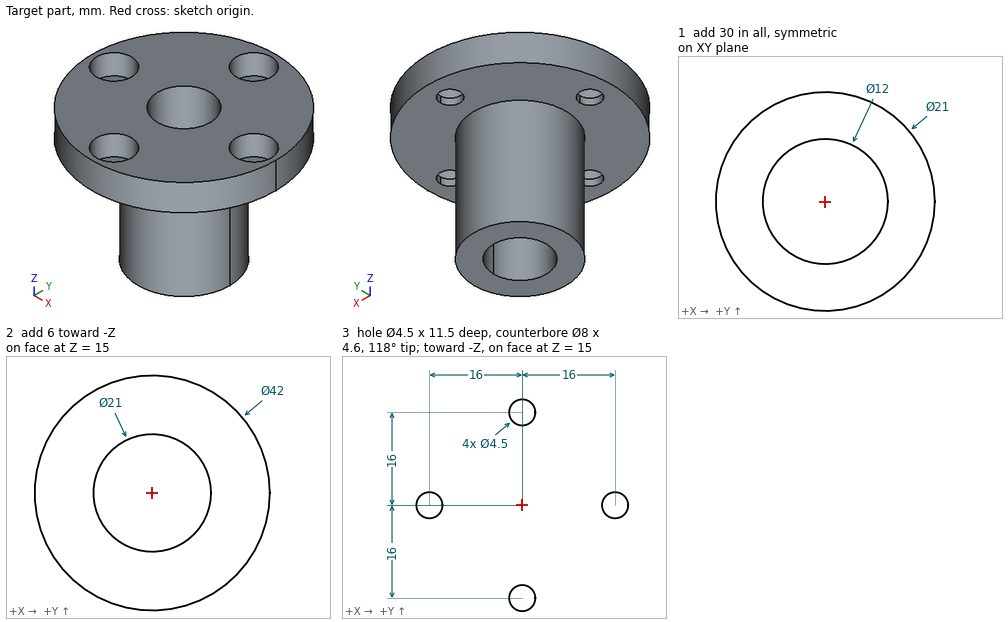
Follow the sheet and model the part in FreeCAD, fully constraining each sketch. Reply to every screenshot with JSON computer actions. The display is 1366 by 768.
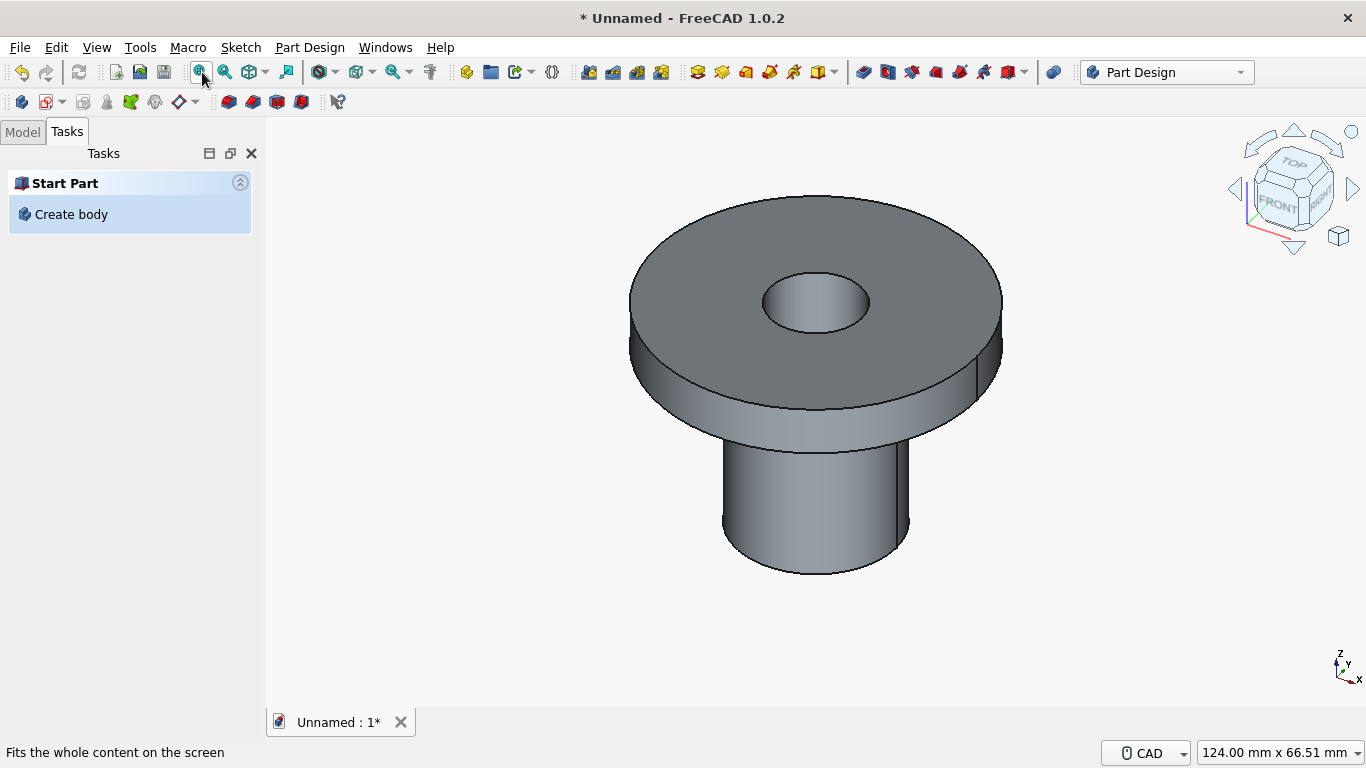
{"action": "left_click", "coordinate": [750, 245]}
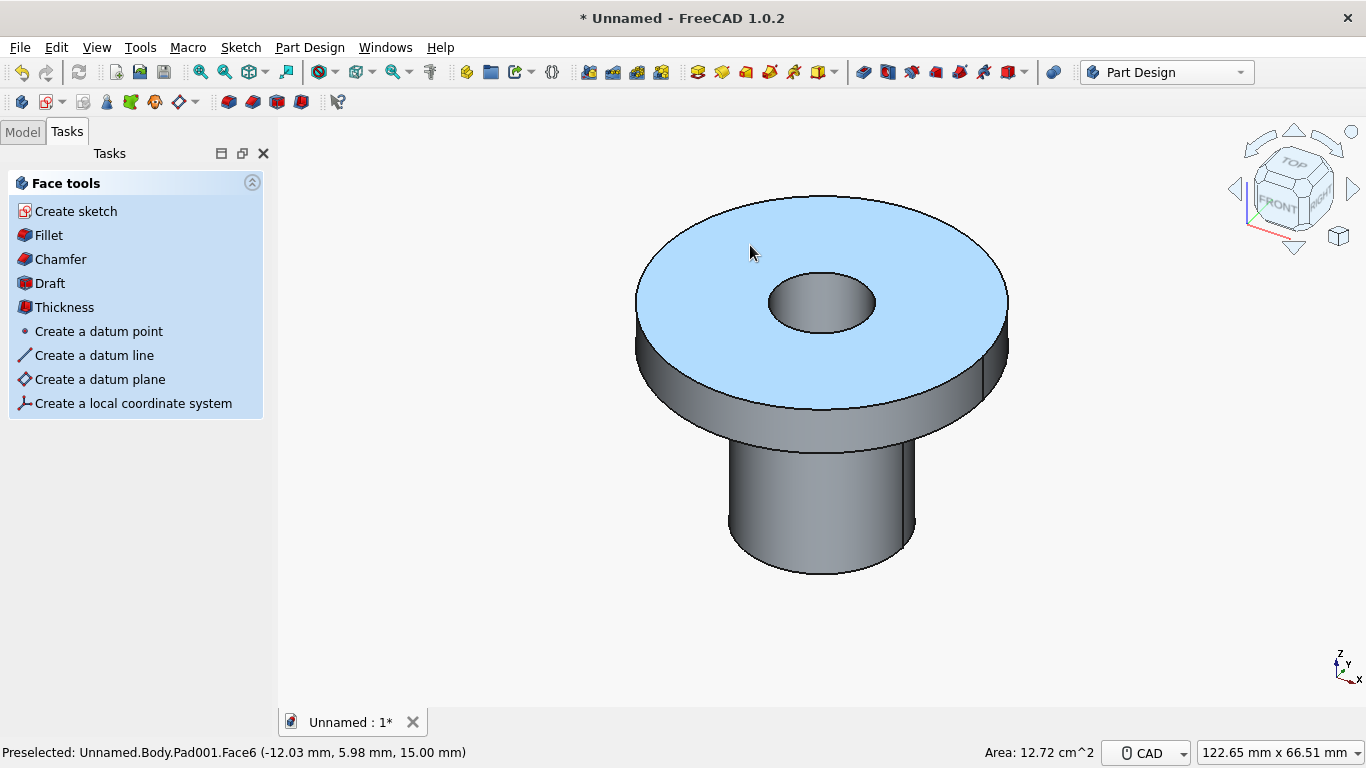
{"action": "left_click", "coordinate": [46, 102]}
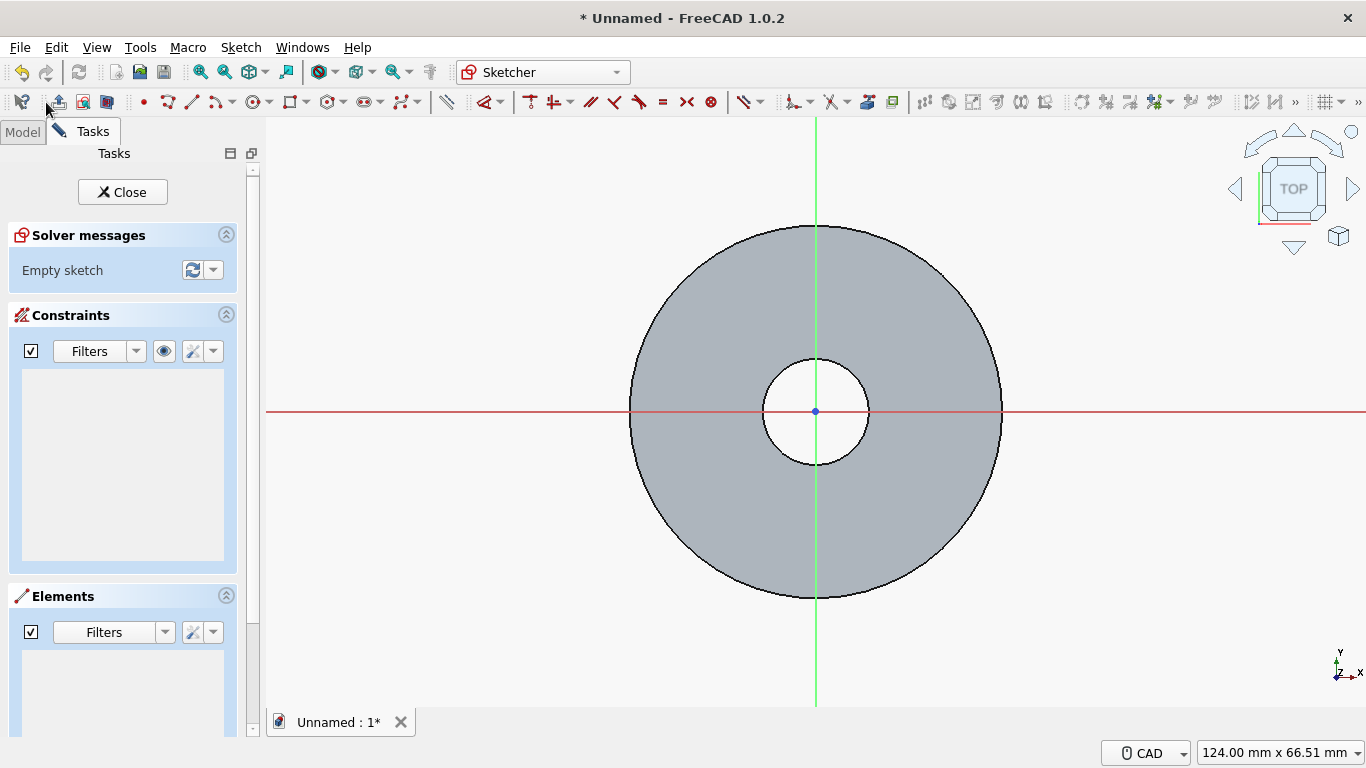
{"action": "left_click", "coordinate": [254, 102]}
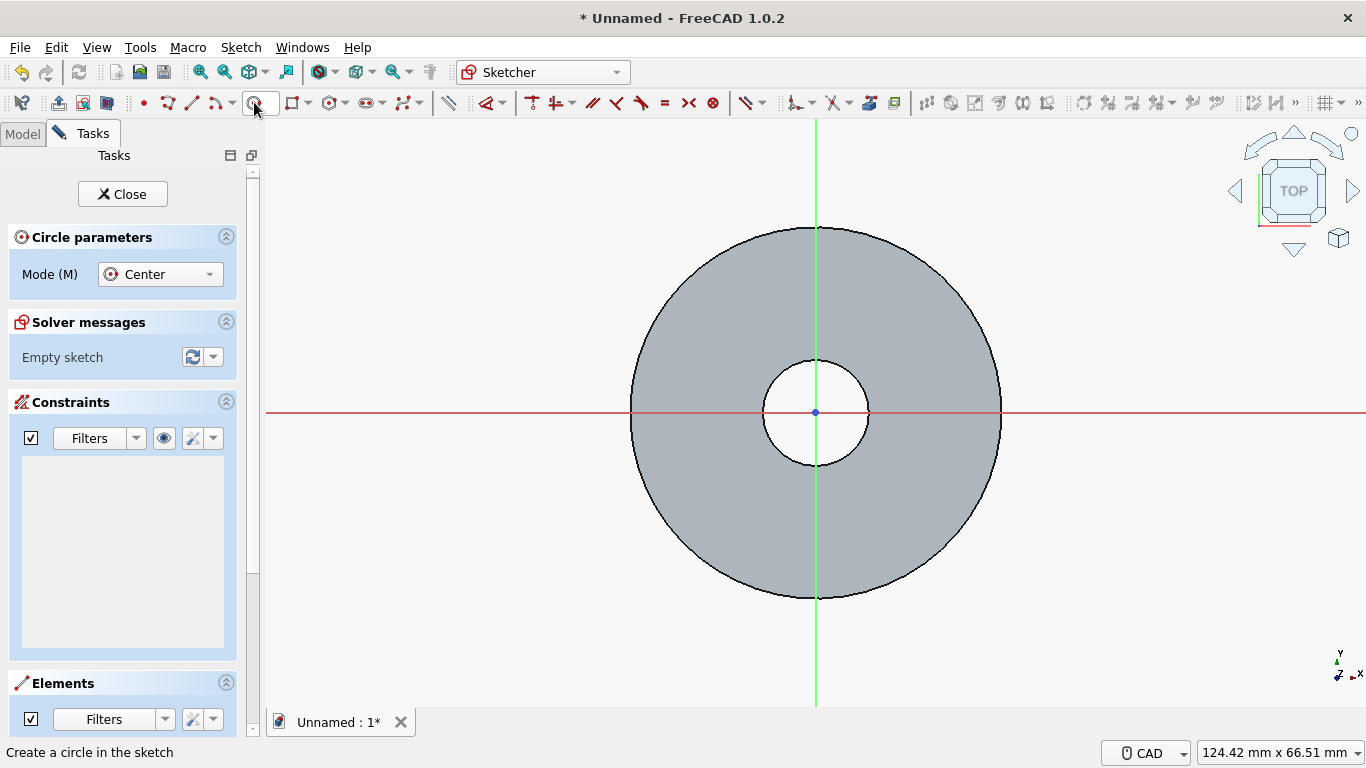
{"action": "left_click", "coordinate": [816, 272]}
{"action": "mouse_move", "coordinate": [830, 257]}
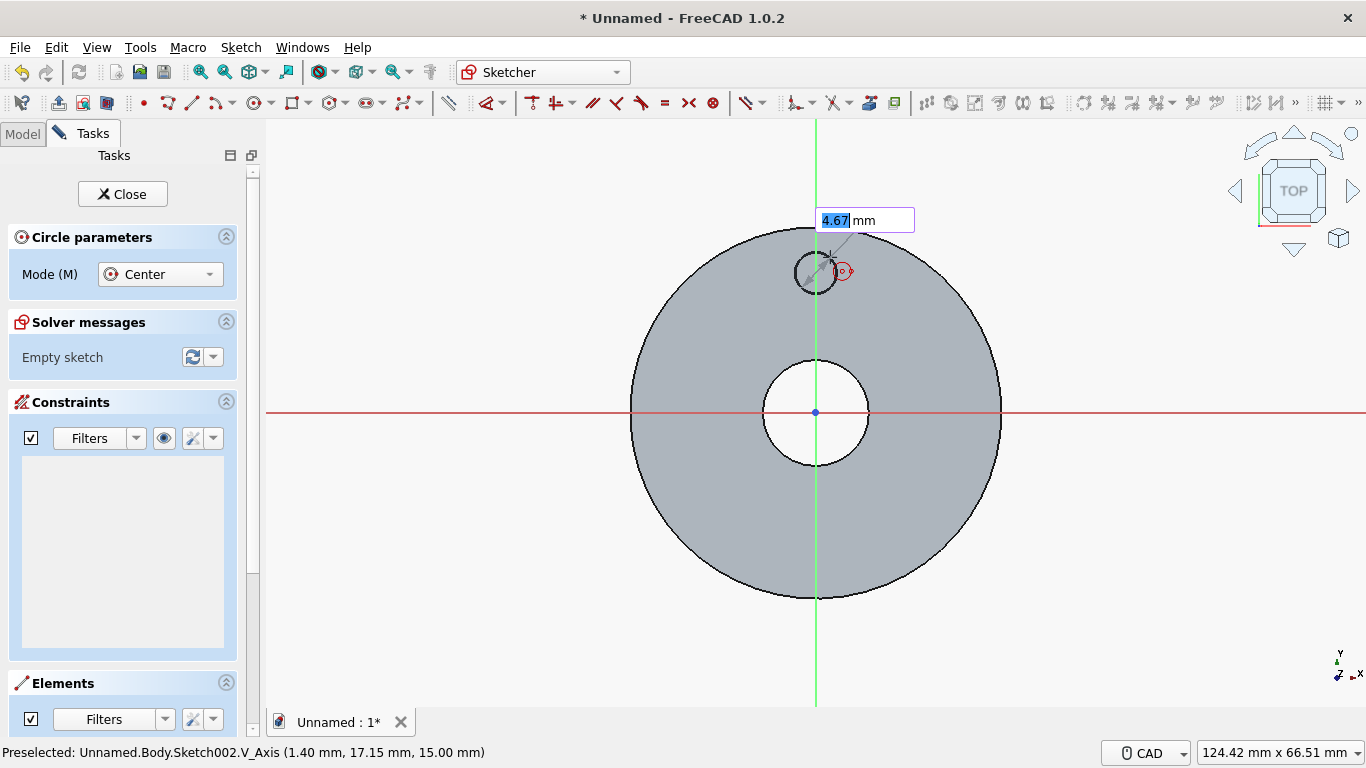
{"action": "type", "text": "4.5"}
{"action": "key", "text": "Return"}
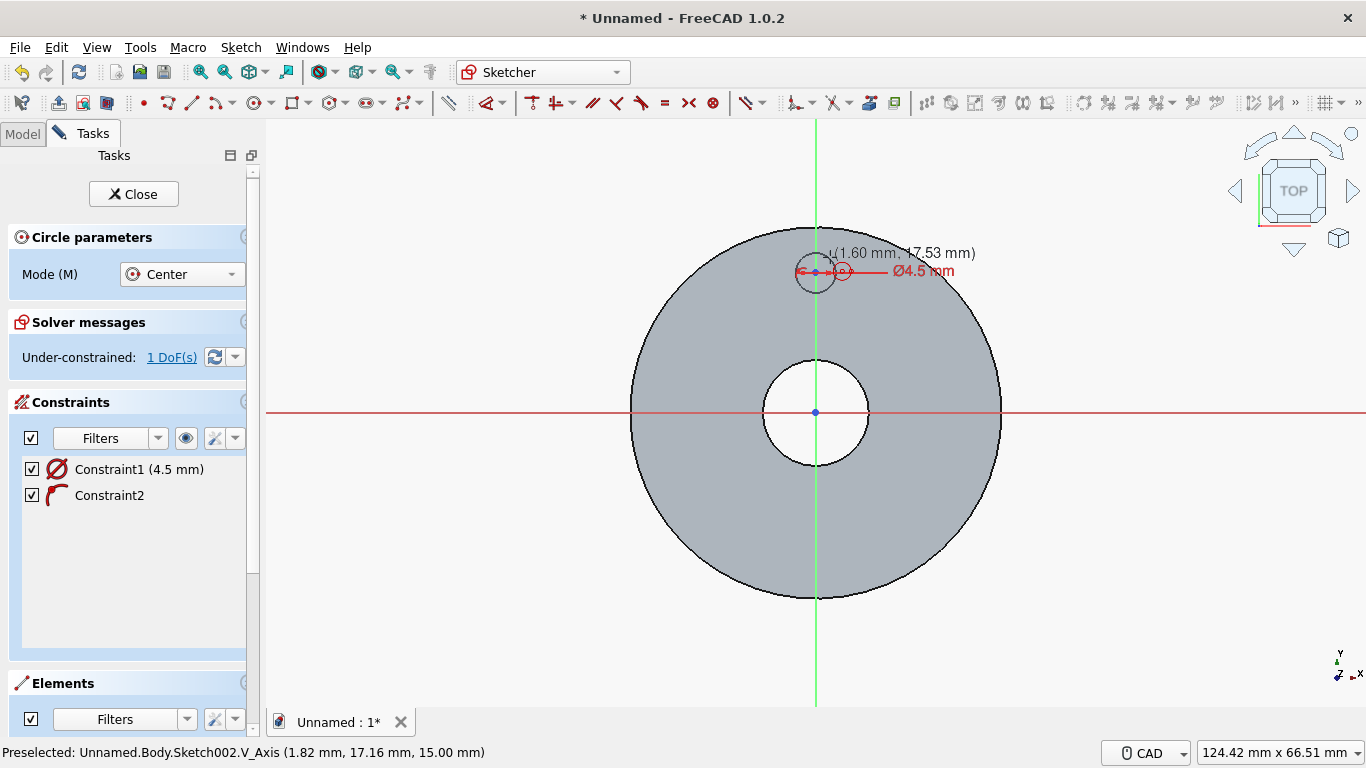
{"action": "left_click", "coordinate": [957, 413]}
{"action": "mouse_move", "coordinate": [971, 399]}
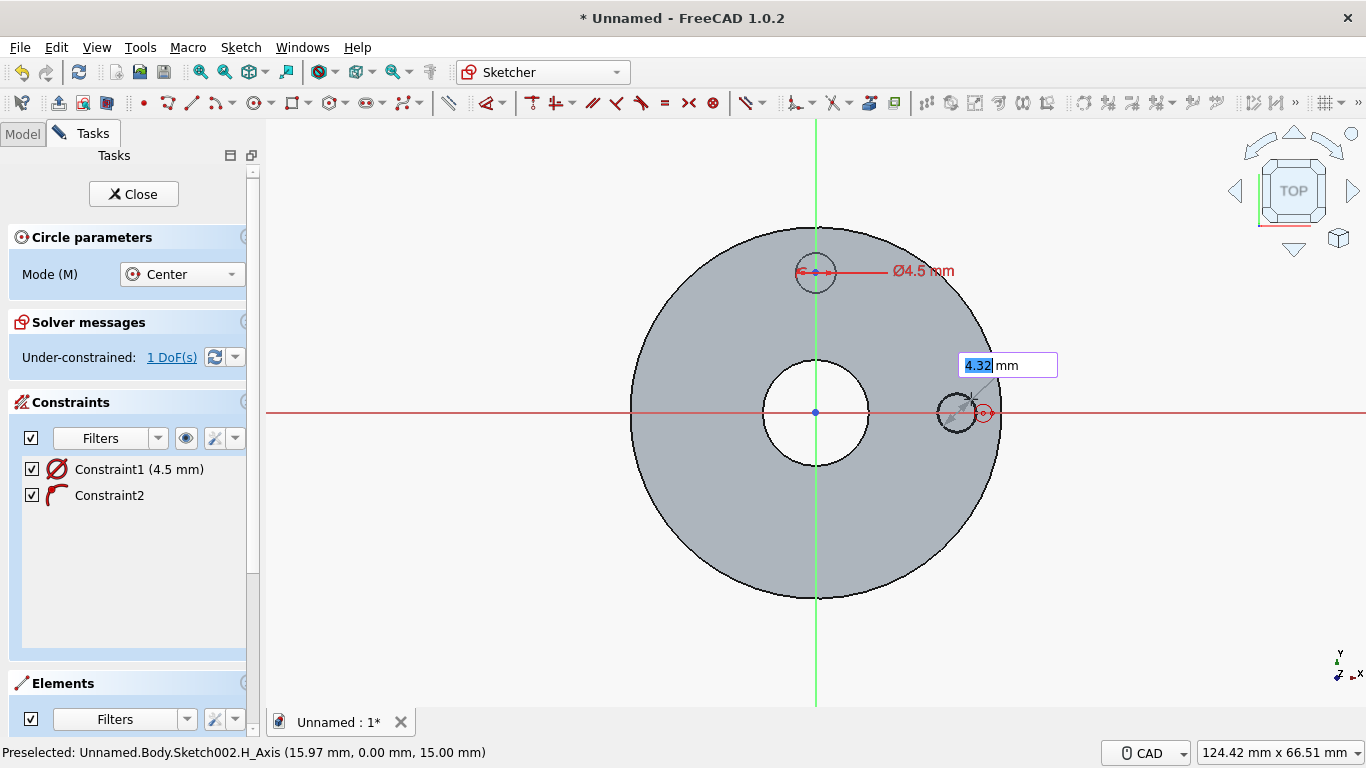
{"action": "type", "text": "4.5"}
{"action": "key", "text": "Return"}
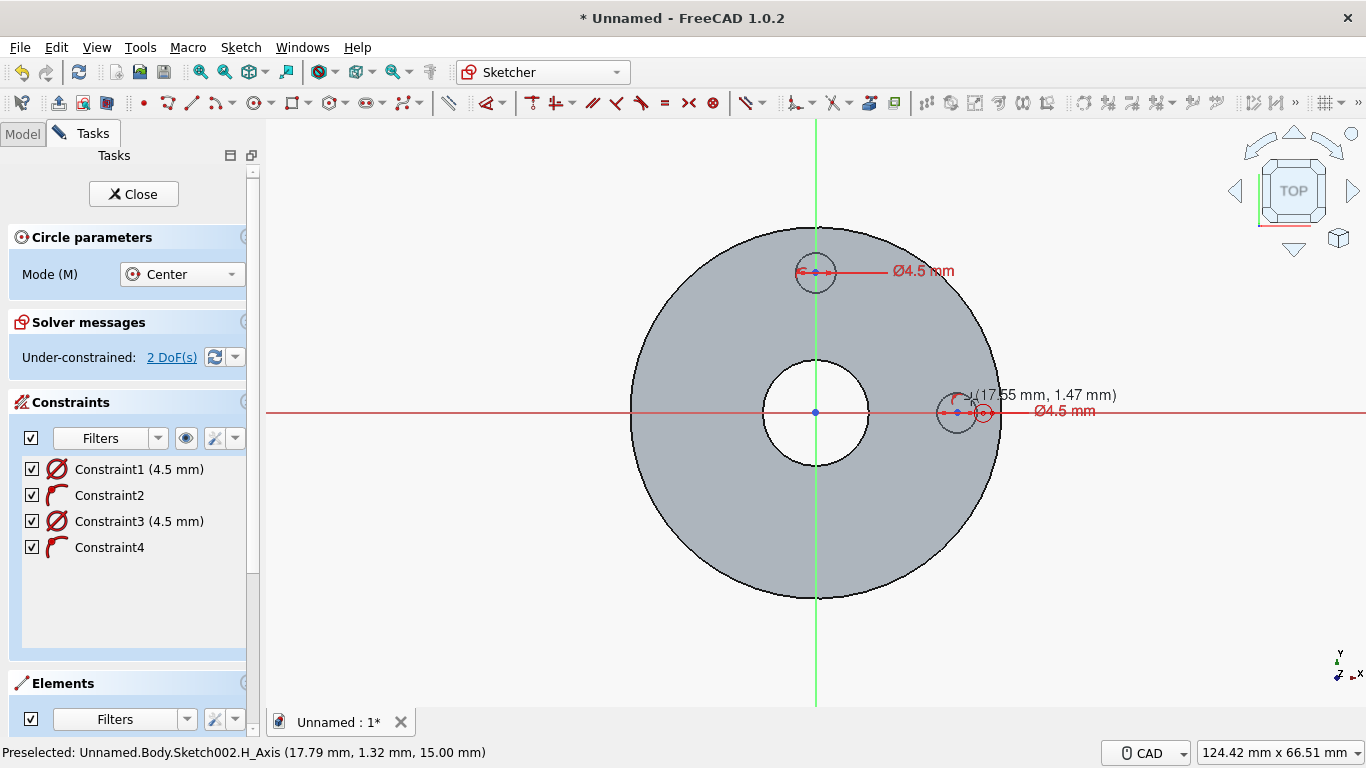
{"action": "left_click", "coordinate": [816, 554]}
{"action": "mouse_move", "coordinate": [830, 540]}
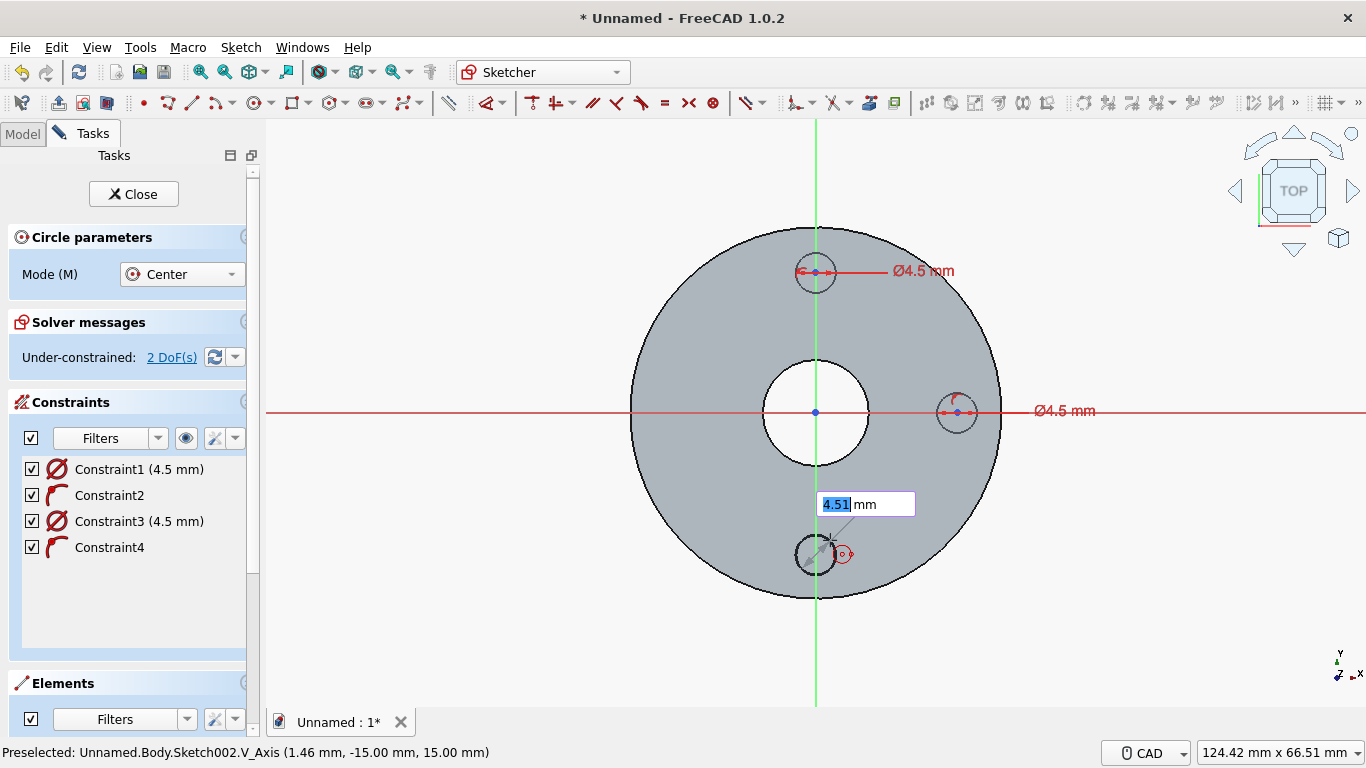
{"action": "type", "text": "4.5"}
{"action": "key", "text": "Return"}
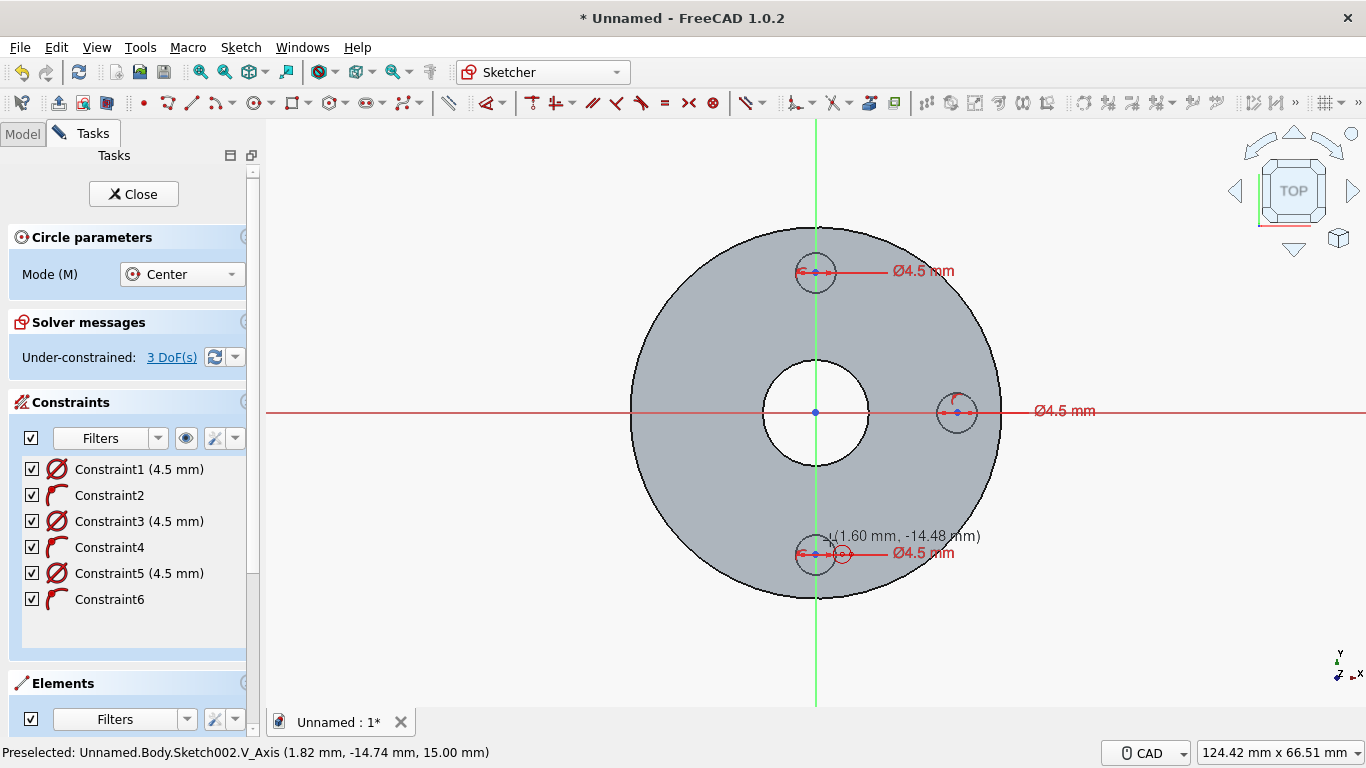
{"action": "left_click", "coordinate": [674, 413]}
{"action": "mouse_move", "coordinate": [688, 399]}